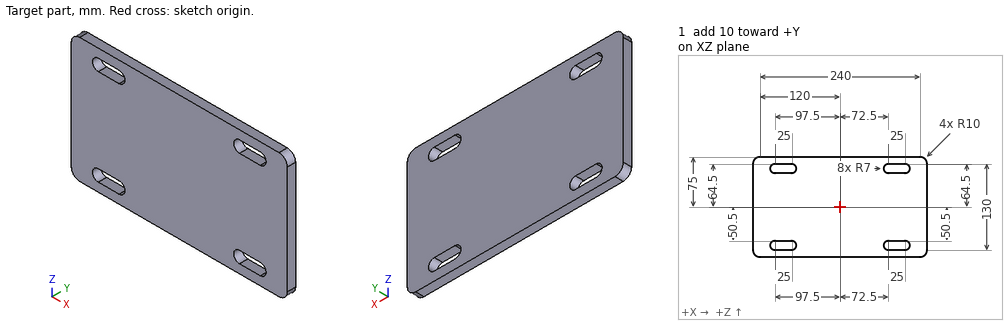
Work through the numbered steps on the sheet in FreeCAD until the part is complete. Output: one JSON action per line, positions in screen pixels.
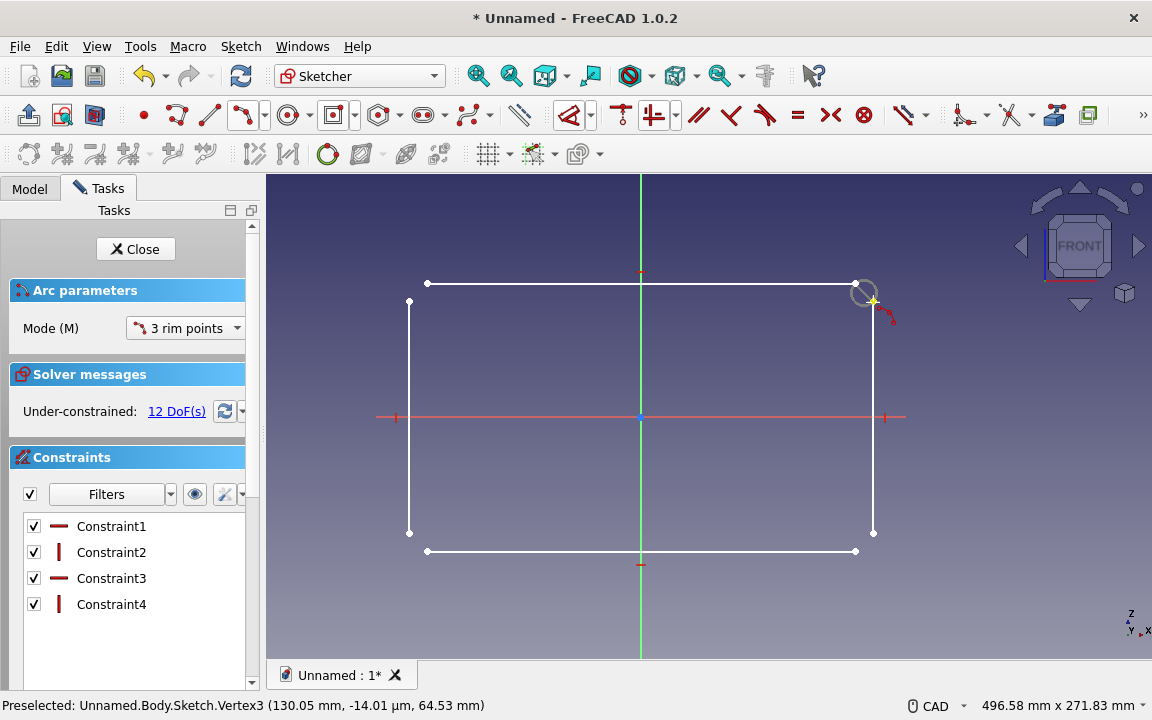
{"action": "scroll", "coordinate": [868, 289], "scroll_direction": "up", "scroll_amount": 6}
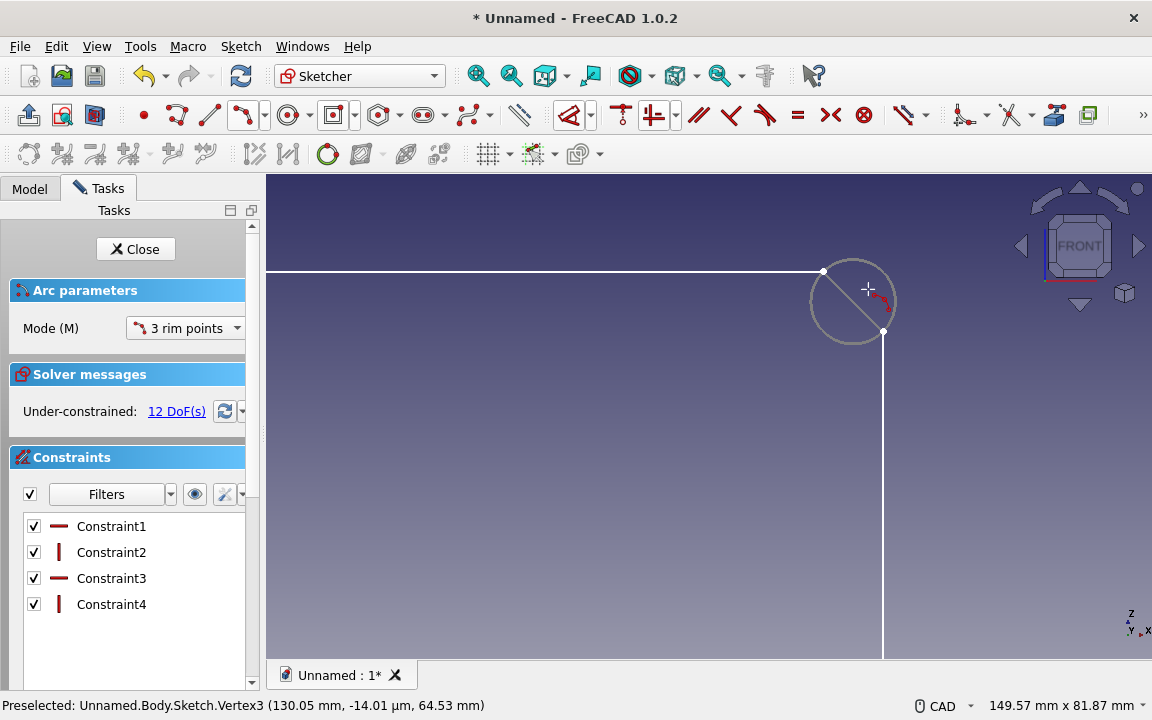
{"action": "left_click", "coordinate": [865, 287]}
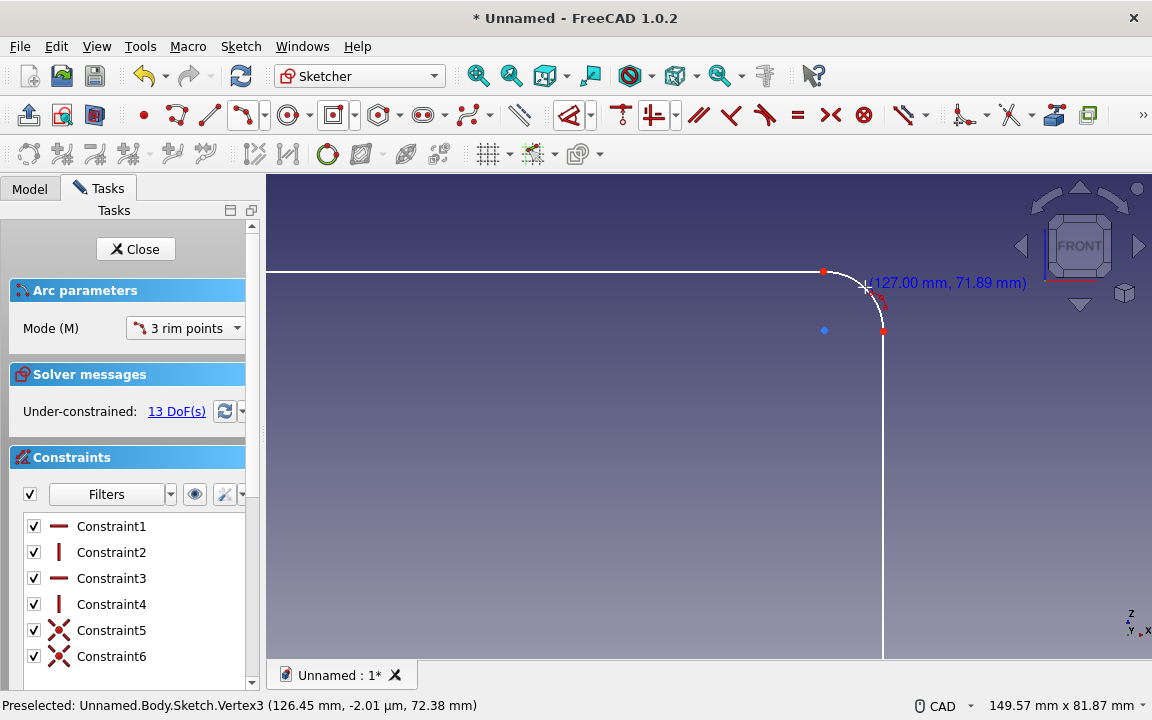
{"action": "scroll", "coordinate": [868, 288], "scroll_direction": "down", "scroll_amount": 6}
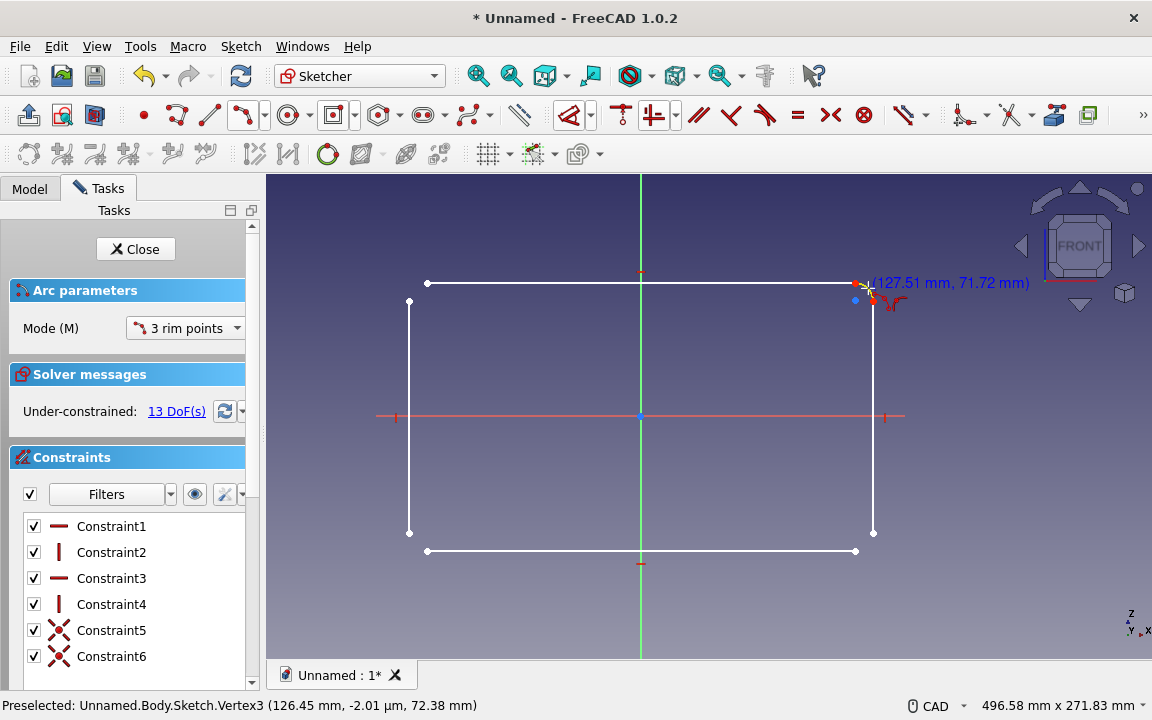
{"action": "left_click", "coordinate": [873, 533]}
{"action": "left_click", "coordinate": [855, 551]}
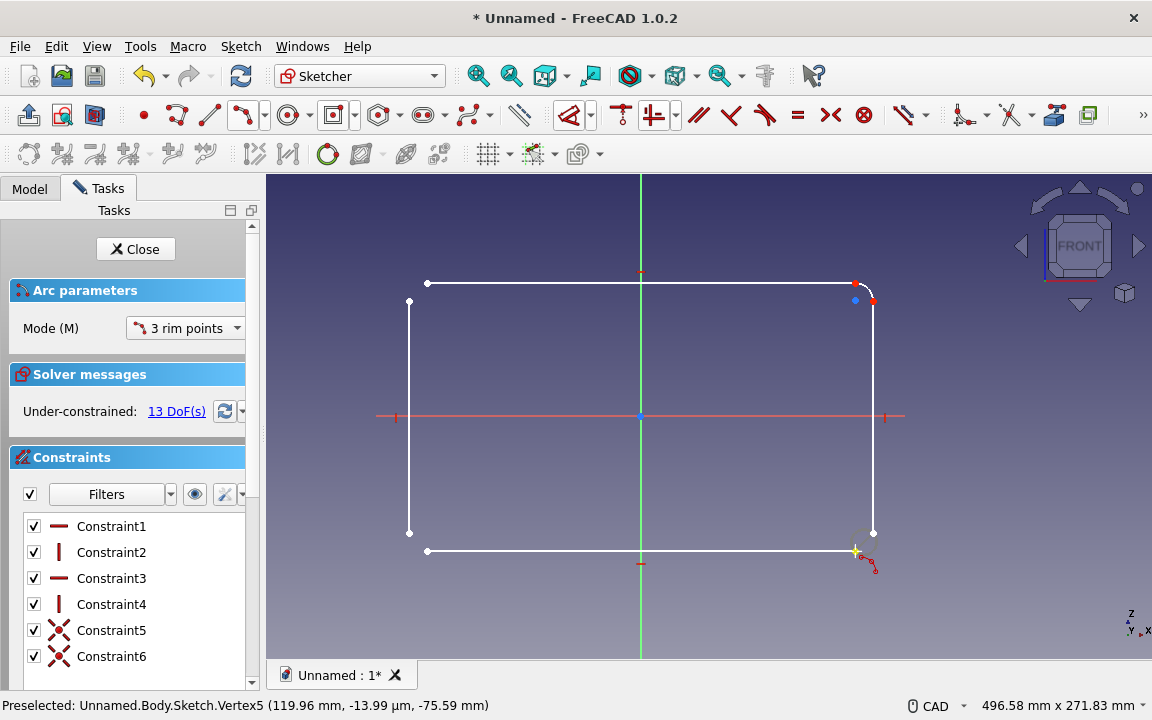
{"action": "scroll", "coordinate": [868, 545], "scroll_direction": "up", "scroll_amount": 6}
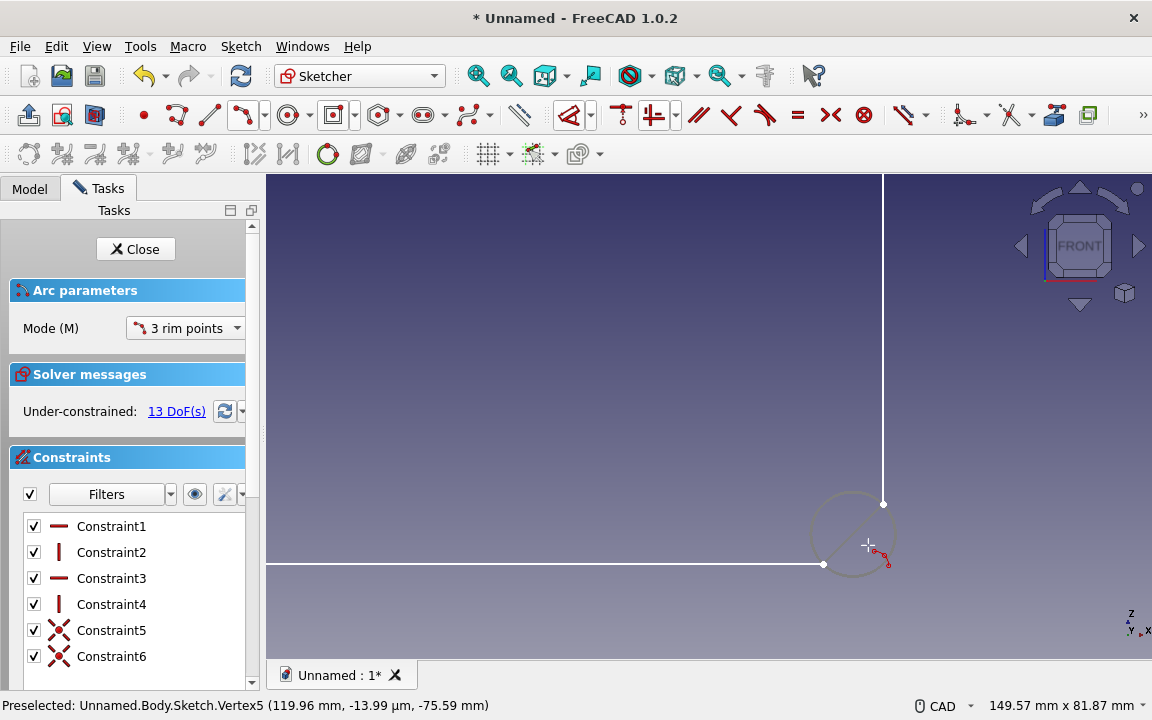
{"action": "left_click", "coordinate": [865, 543]}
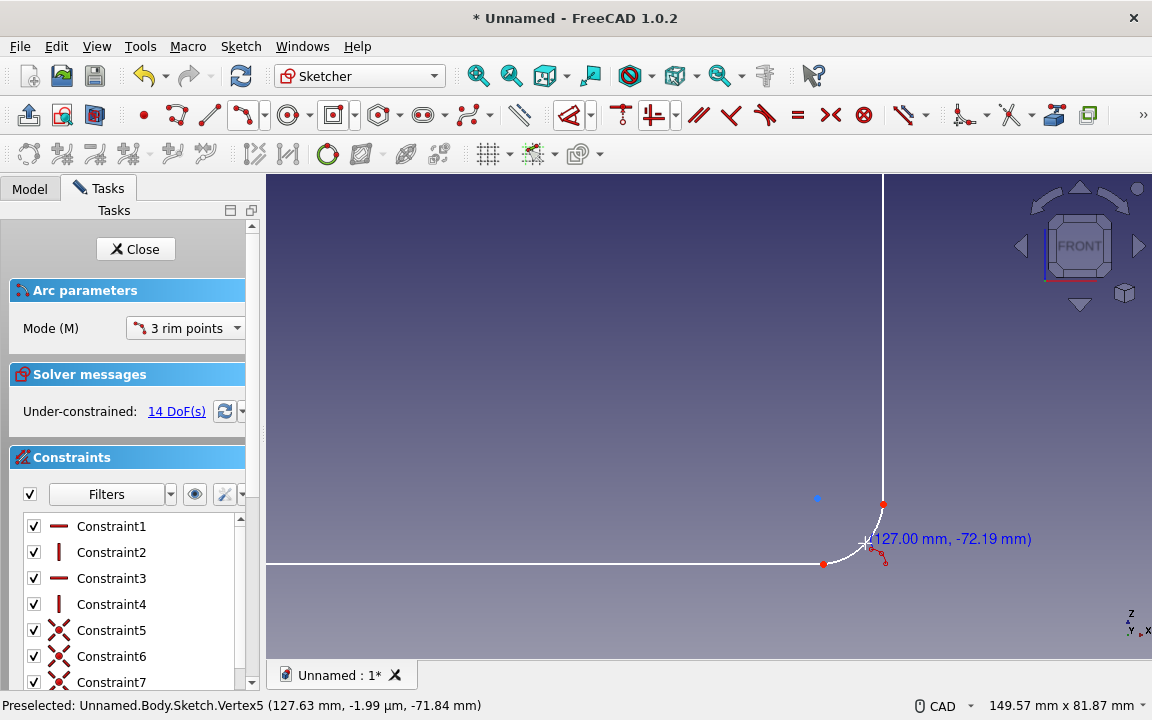
{"action": "scroll", "coordinate": [868, 546], "scroll_direction": "down", "scroll_amount": 6}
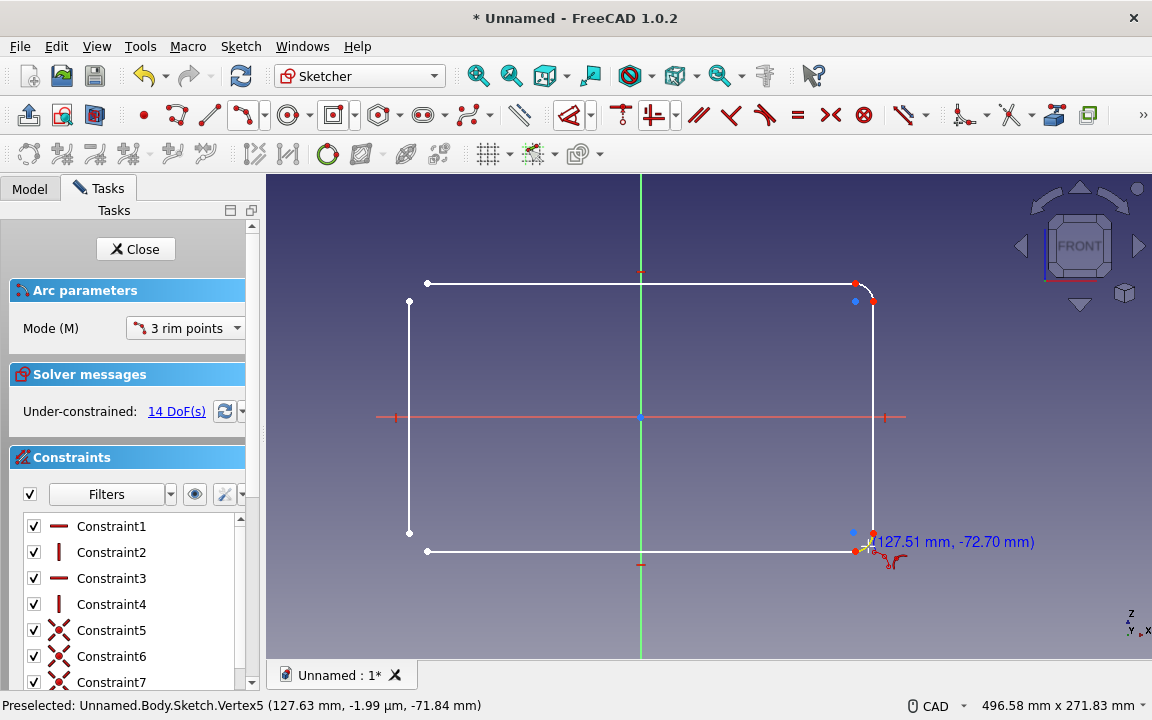
{"action": "left_click", "coordinate": [427, 552]}
{"action": "left_click", "coordinate": [409, 534]}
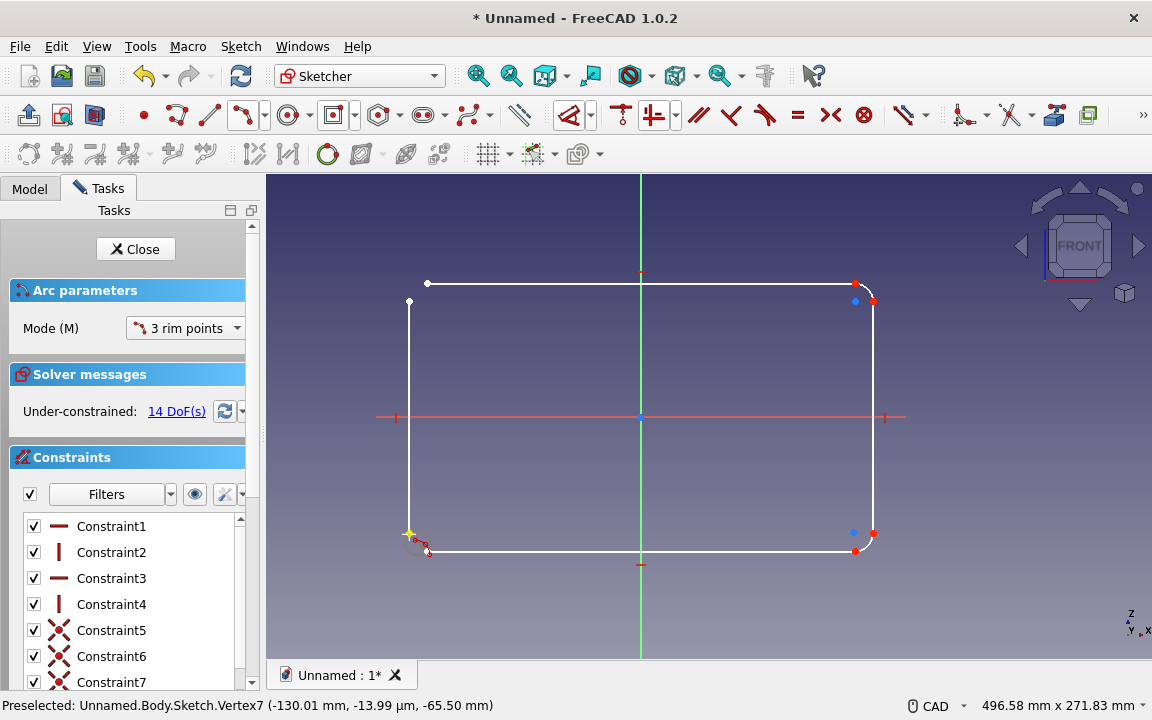
{"action": "scroll", "coordinate": [414, 546], "scroll_direction": "up", "scroll_amount": 6}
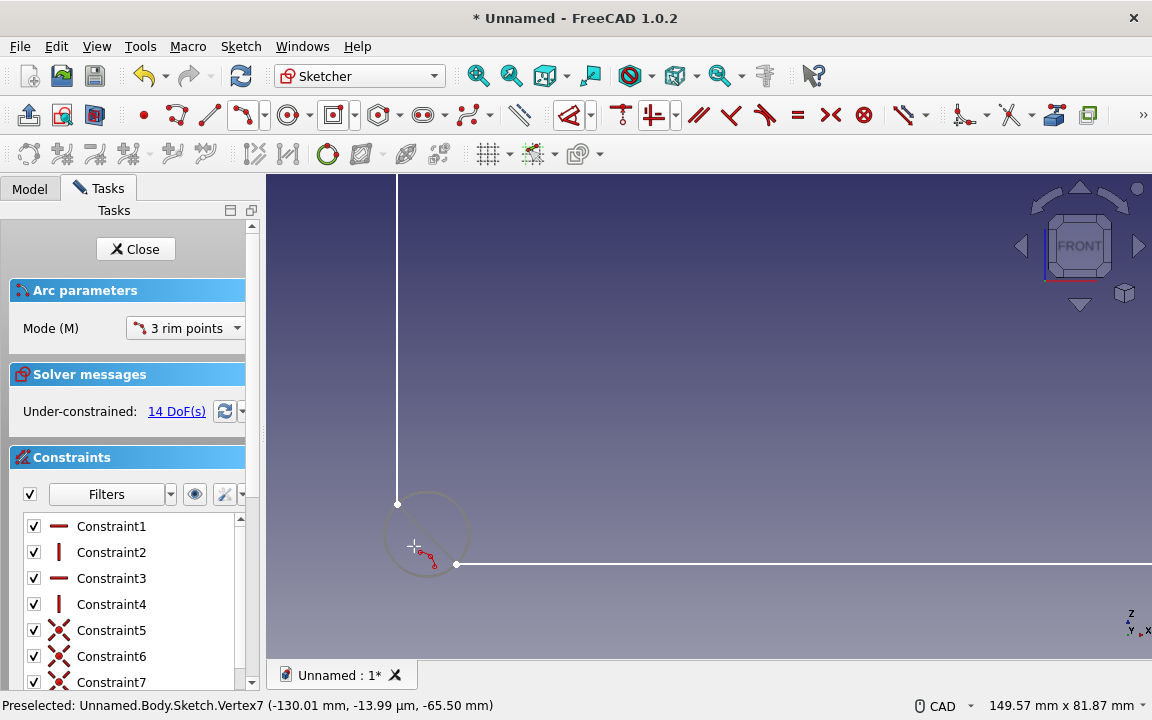
{"action": "left_click", "coordinate": [414, 543]}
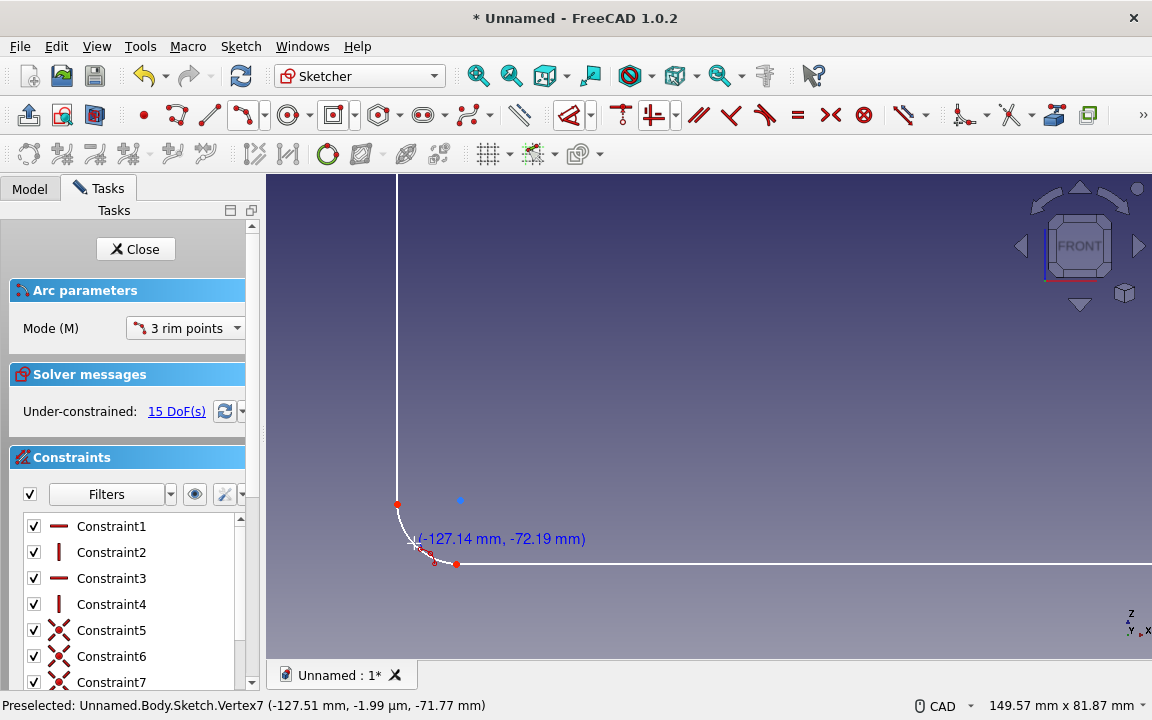
{"action": "scroll", "coordinate": [413, 546], "scroll_direction": "down", "scroll_amount": 6}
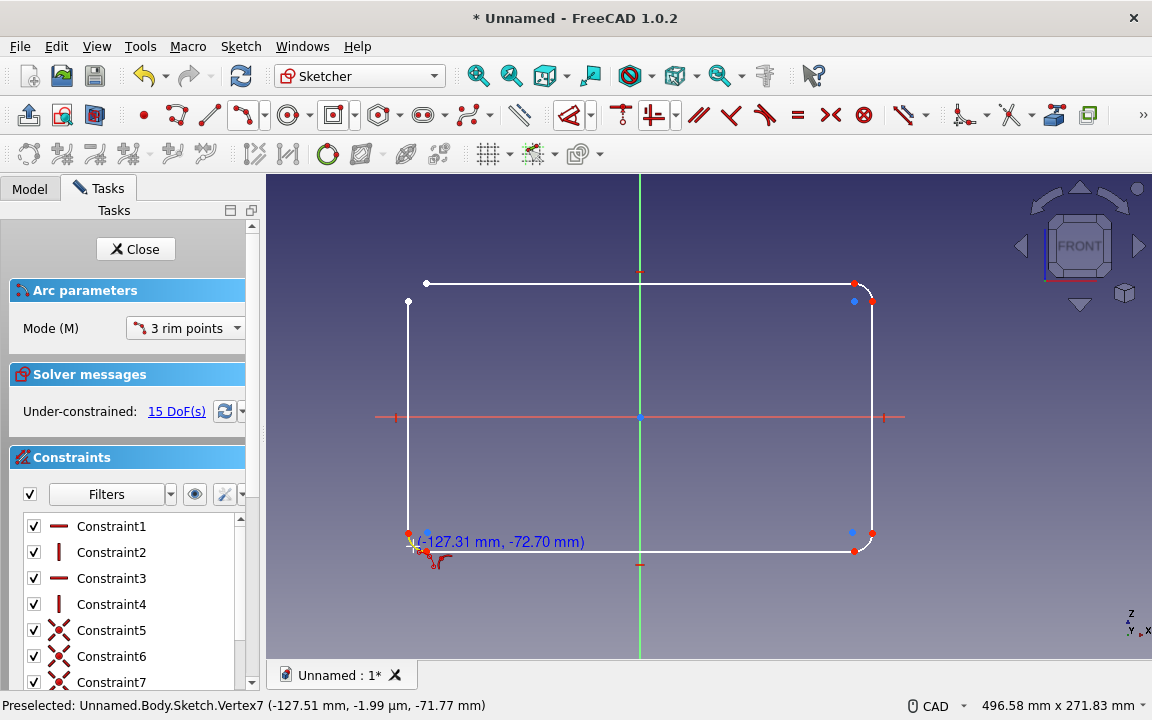
{"action": "left_click", "coordinate": [408, 302]}
{"action": "left_click", "coordinate": [426, 284]}